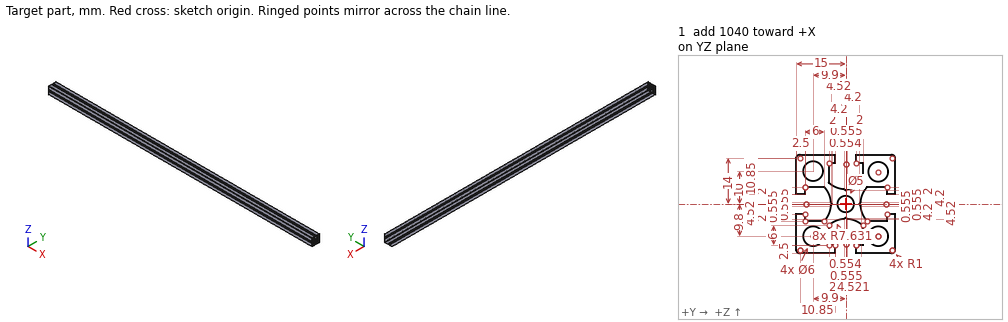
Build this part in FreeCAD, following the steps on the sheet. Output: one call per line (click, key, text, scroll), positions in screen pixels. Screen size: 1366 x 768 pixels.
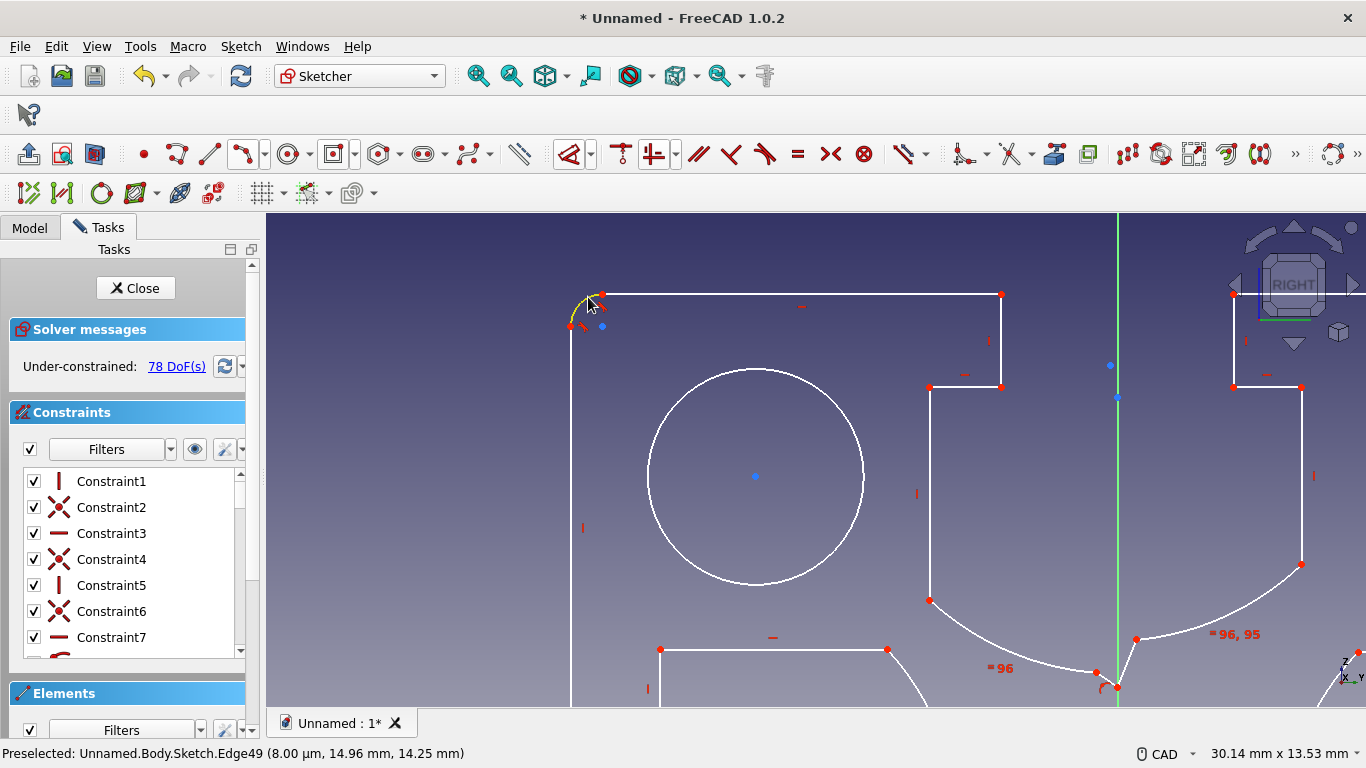
click(588, 298)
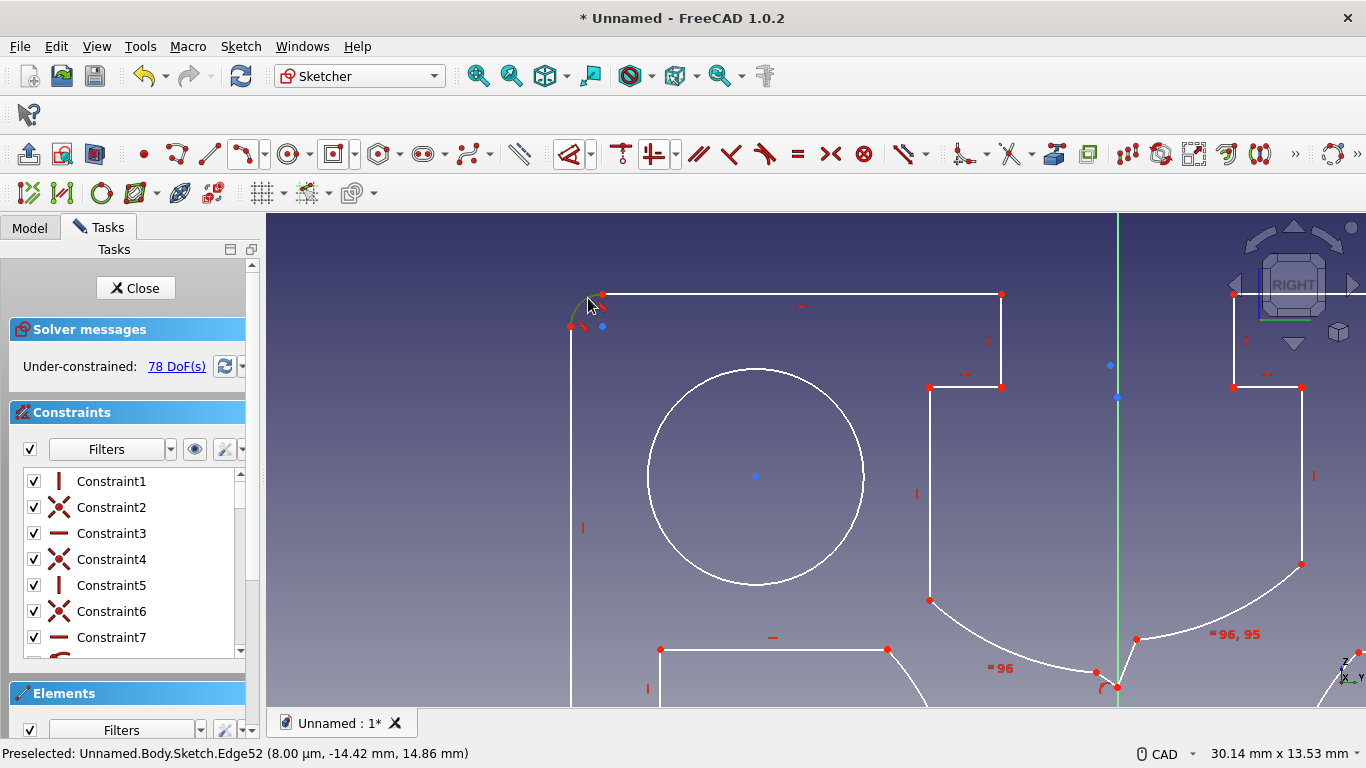
click(798, 154)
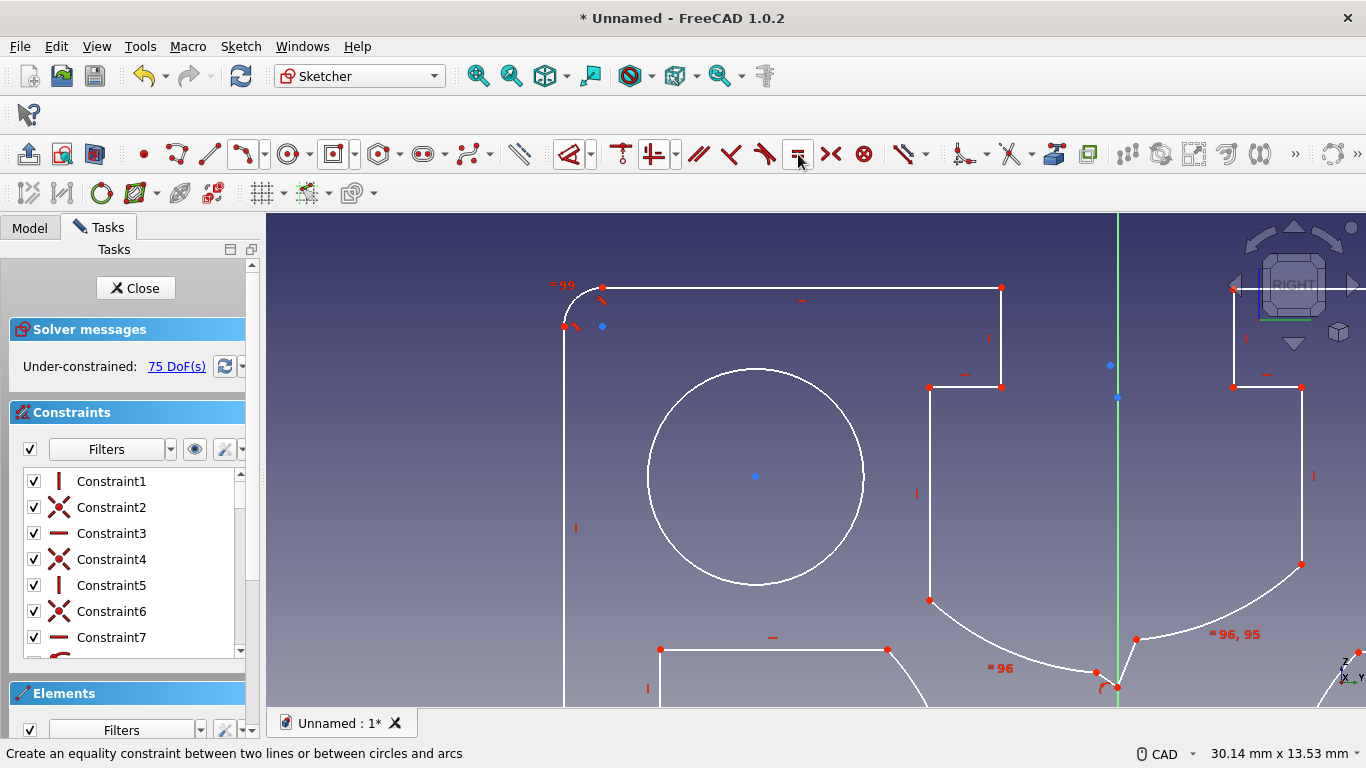
click(832, 400)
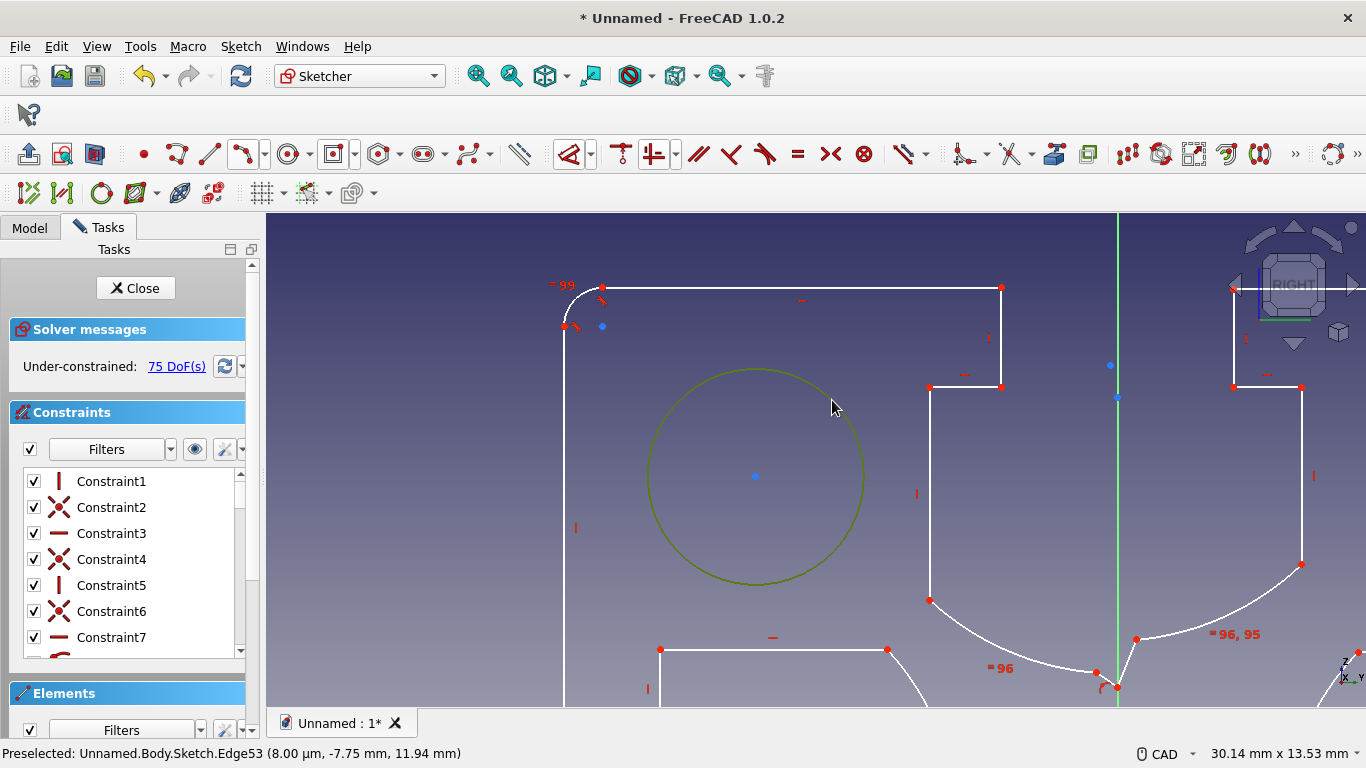
scroll(588, 297, down, 6)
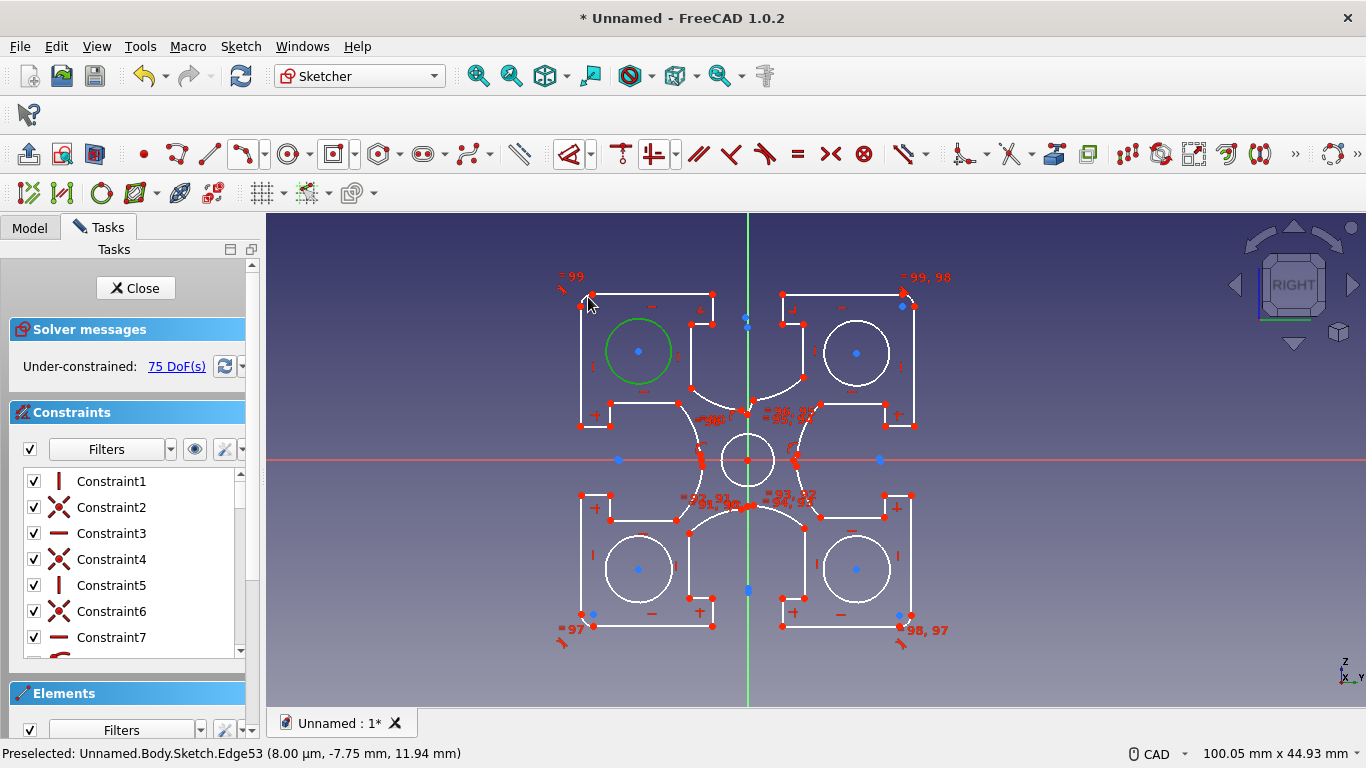
click(662, 546)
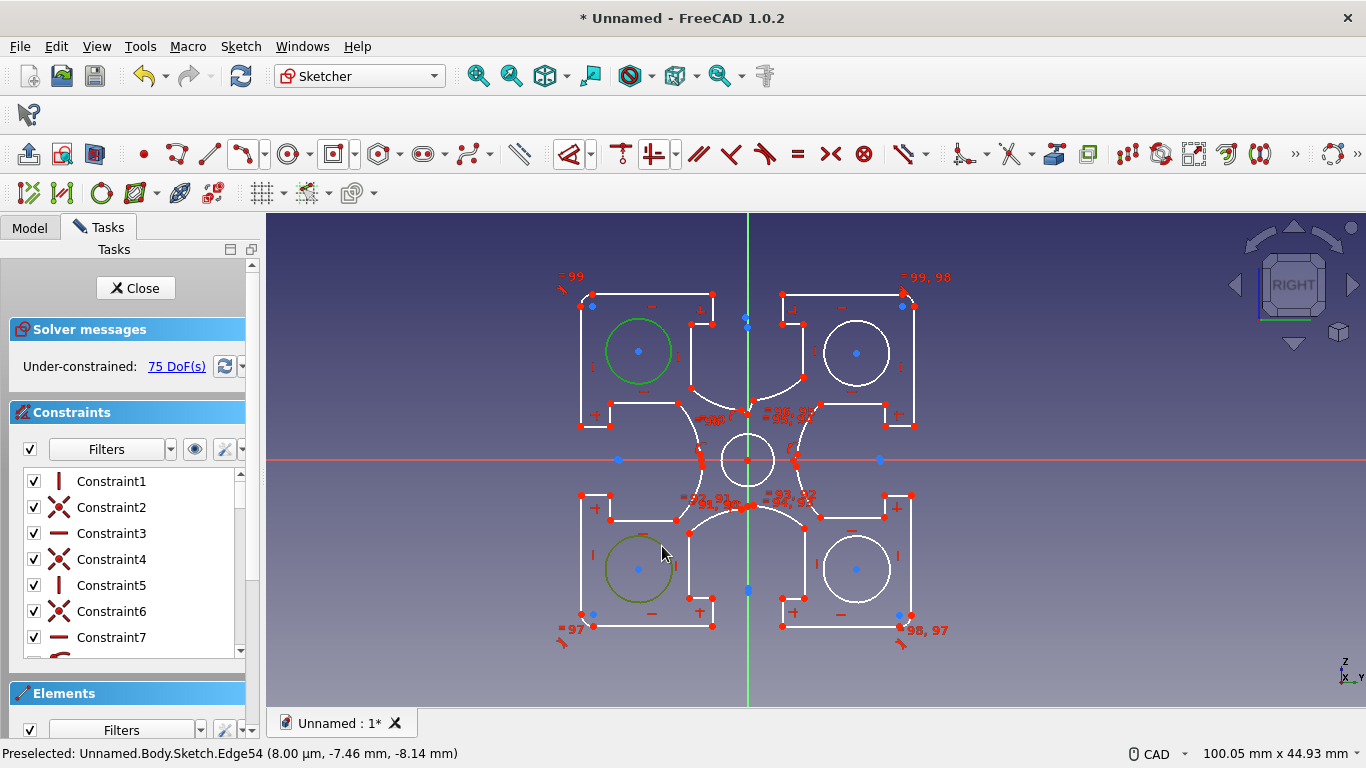
click(880, 330)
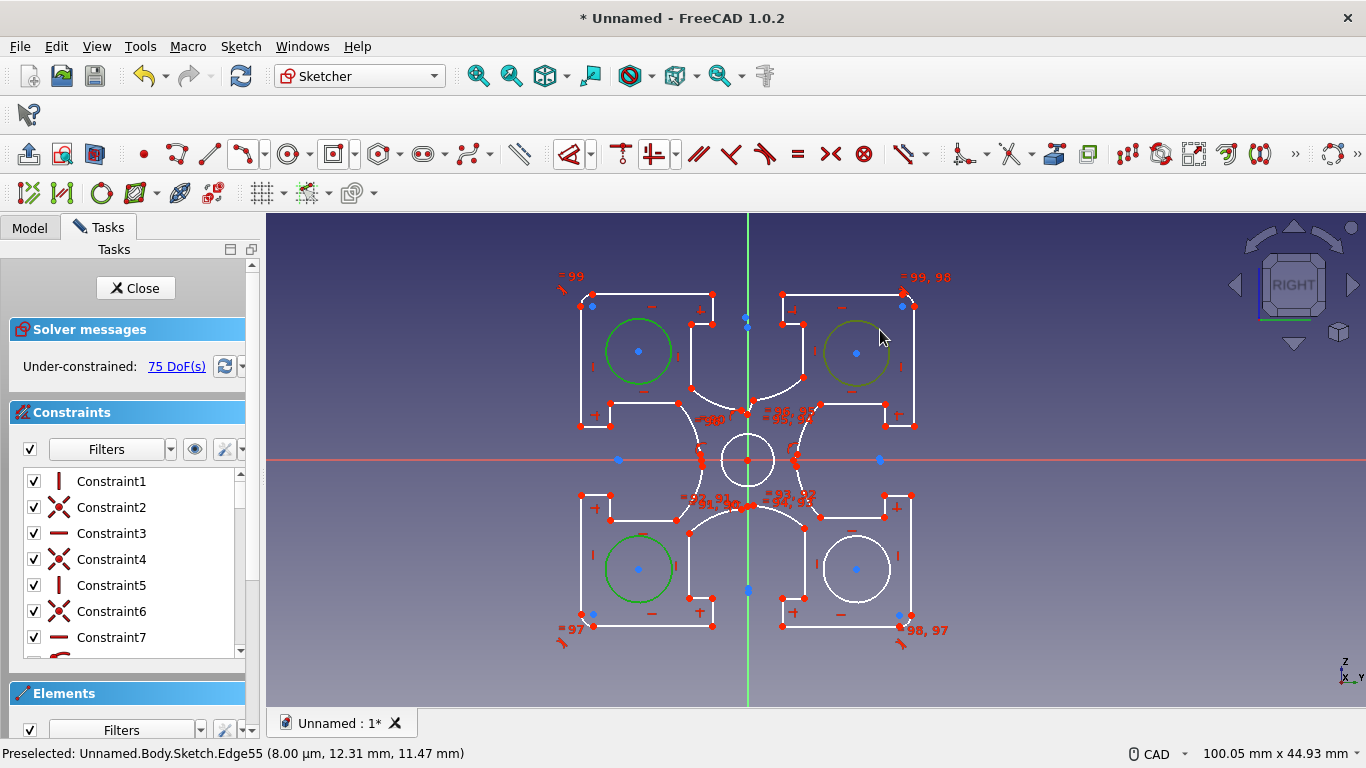
click(880, 546)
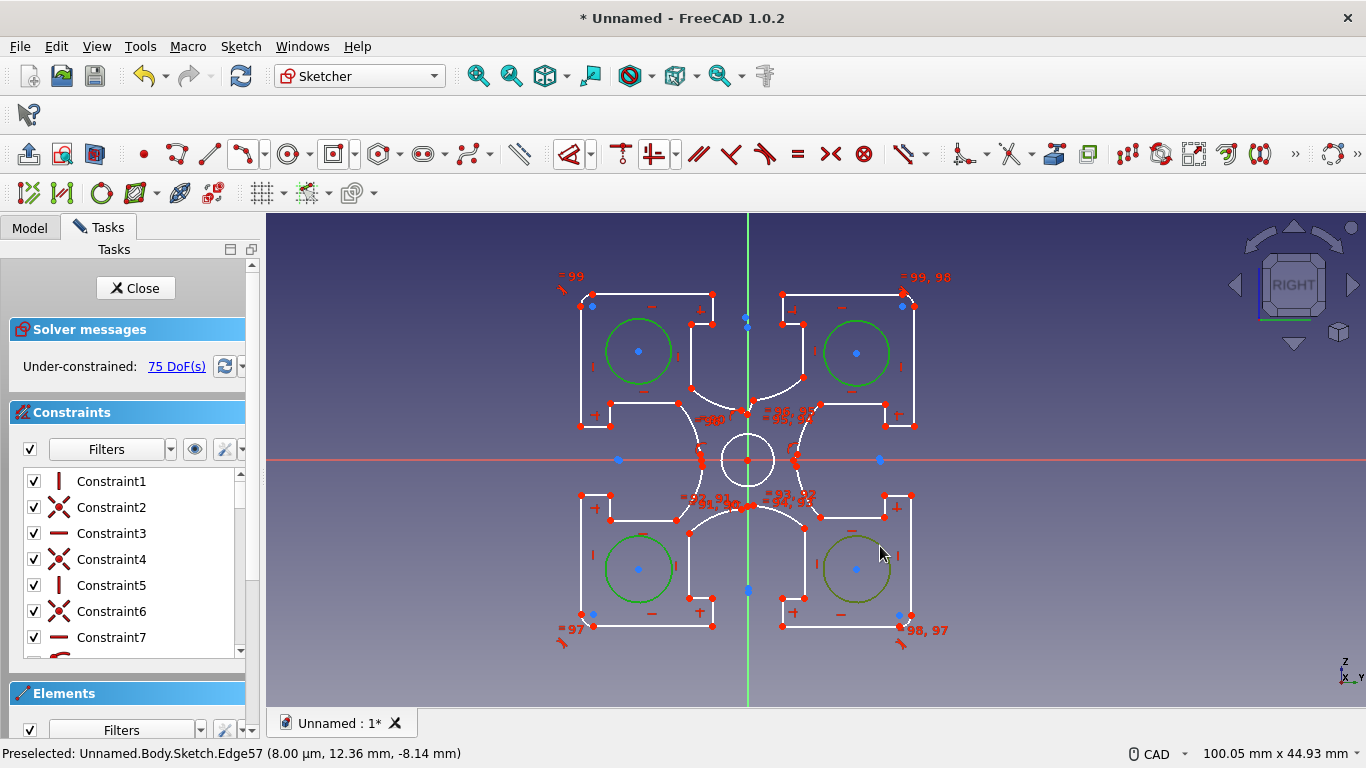
key(e)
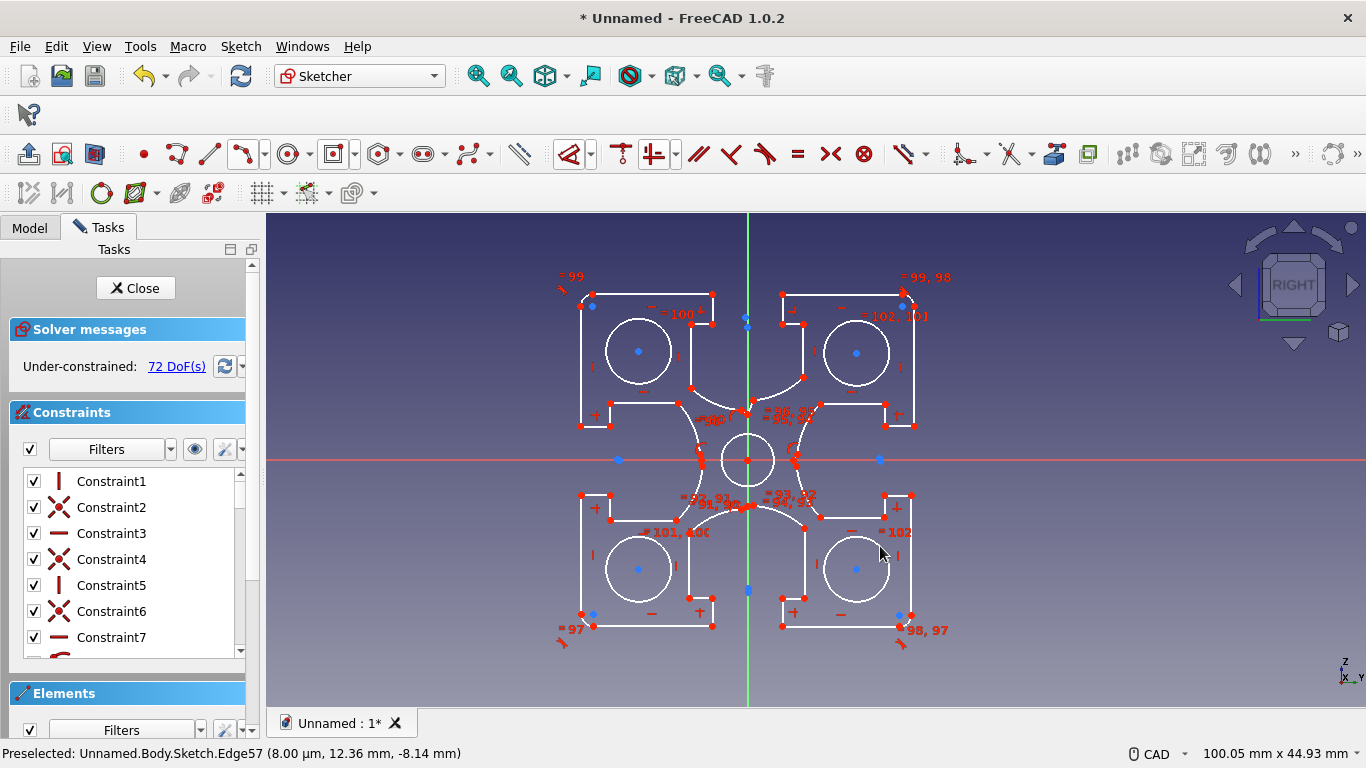
scroll(617, 459, up, 8)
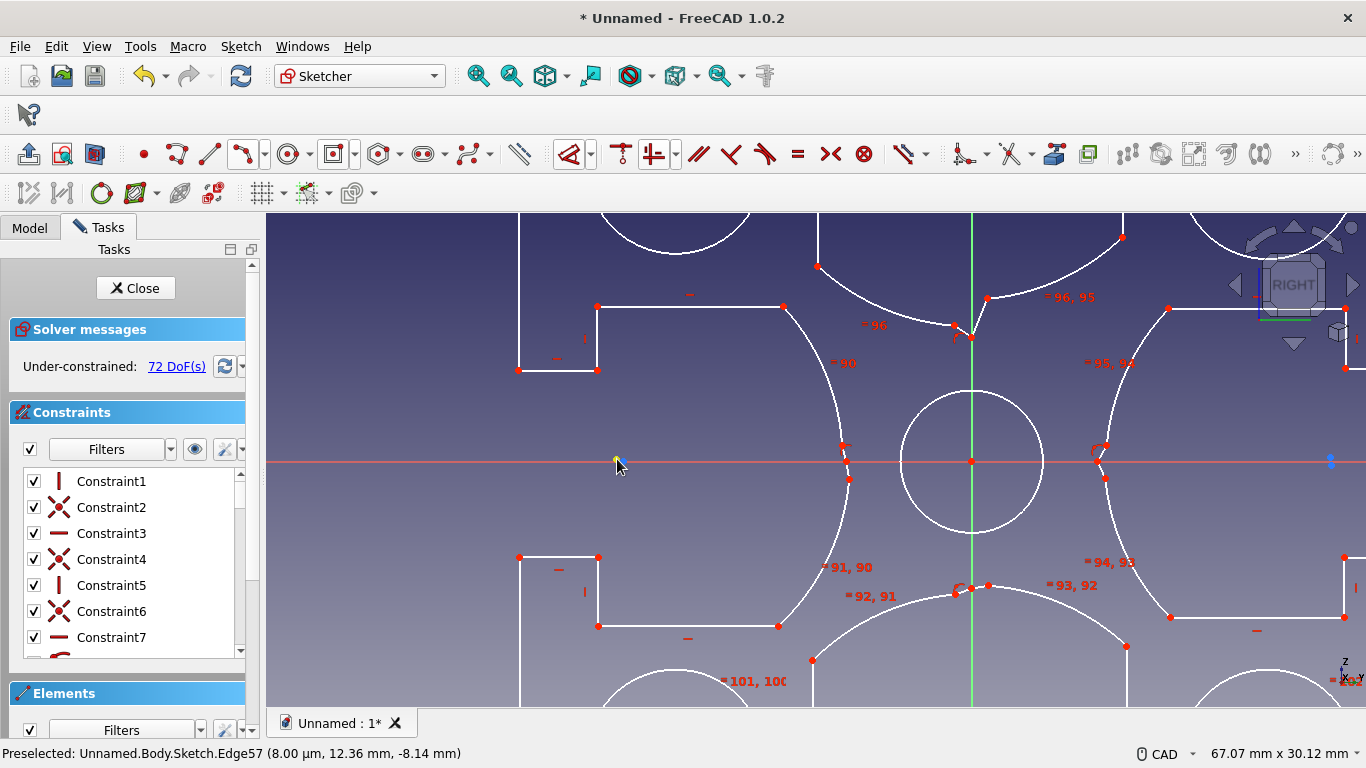
click(616, 459)